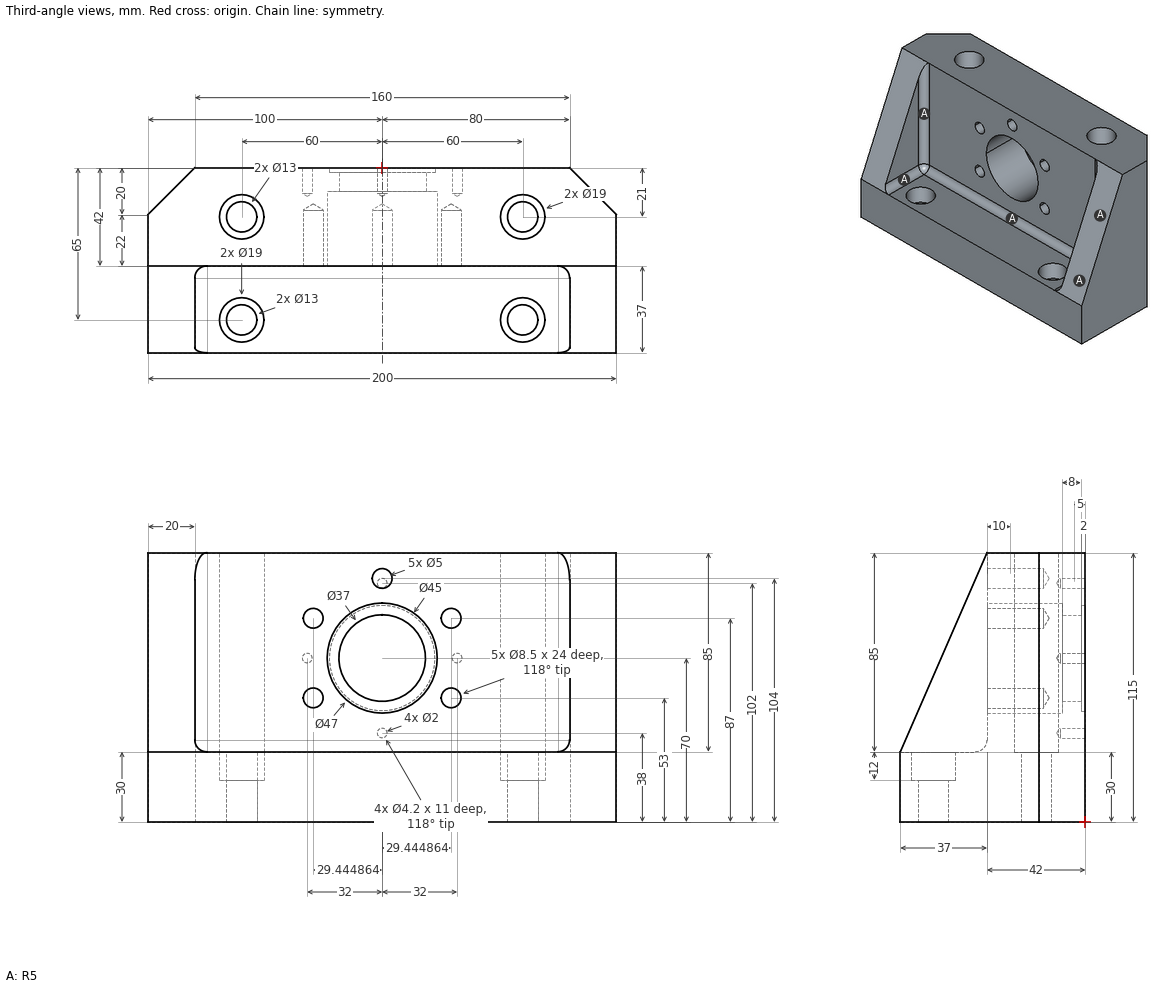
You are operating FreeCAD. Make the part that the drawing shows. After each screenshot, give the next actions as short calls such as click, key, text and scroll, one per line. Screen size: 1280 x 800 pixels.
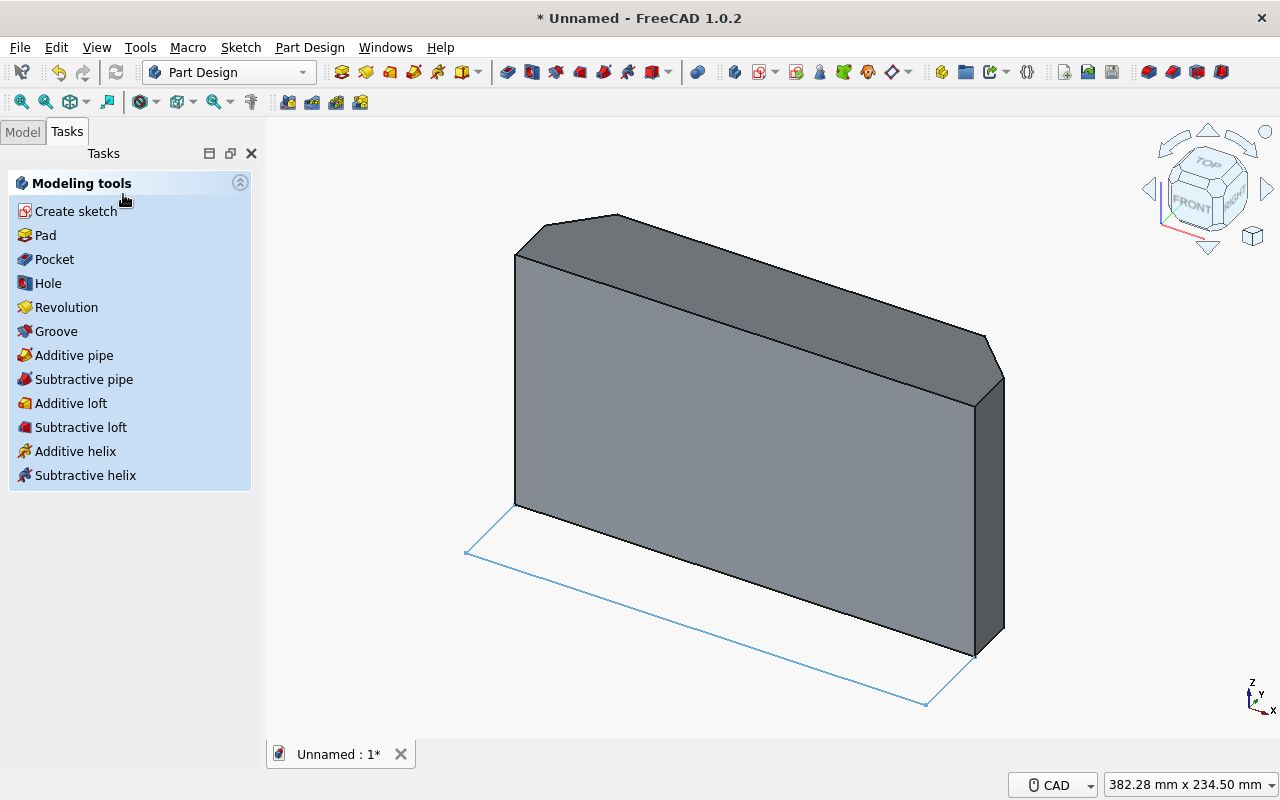
click(342, 72)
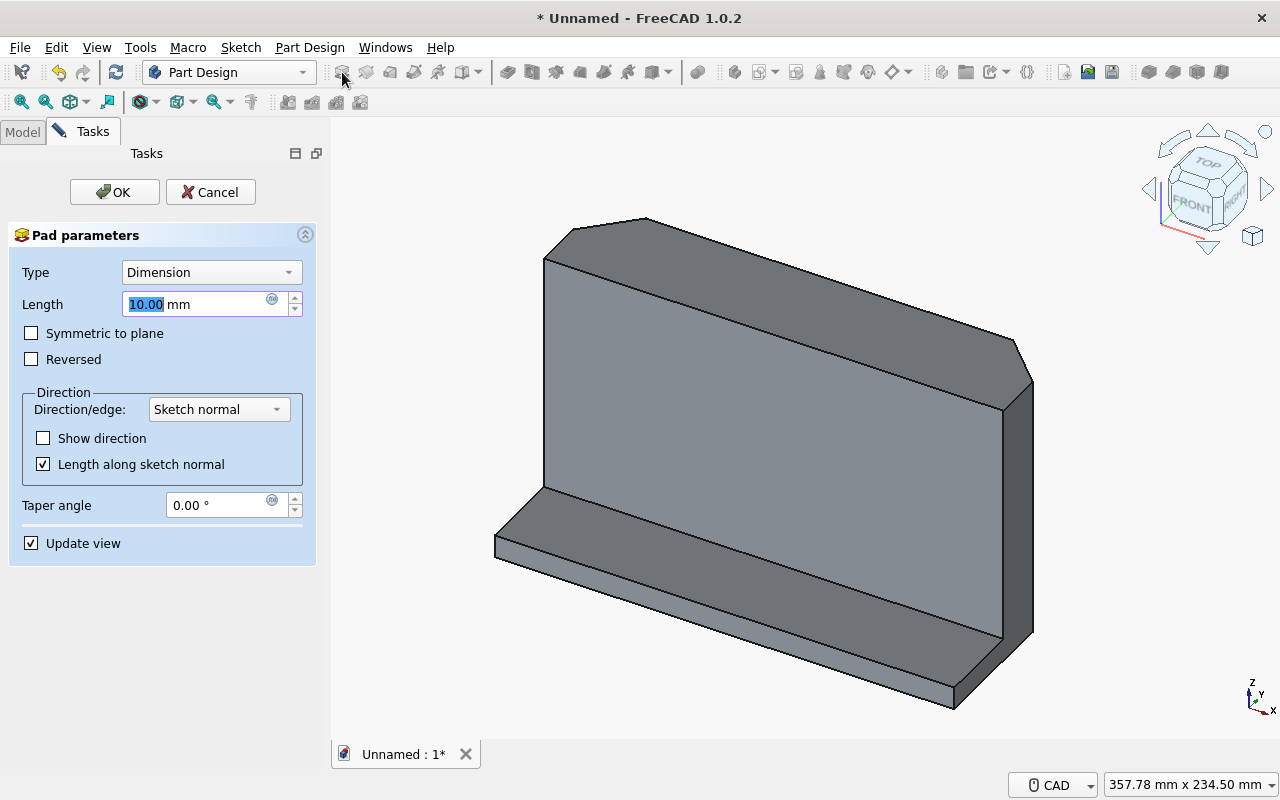
text(30)
key(Tab)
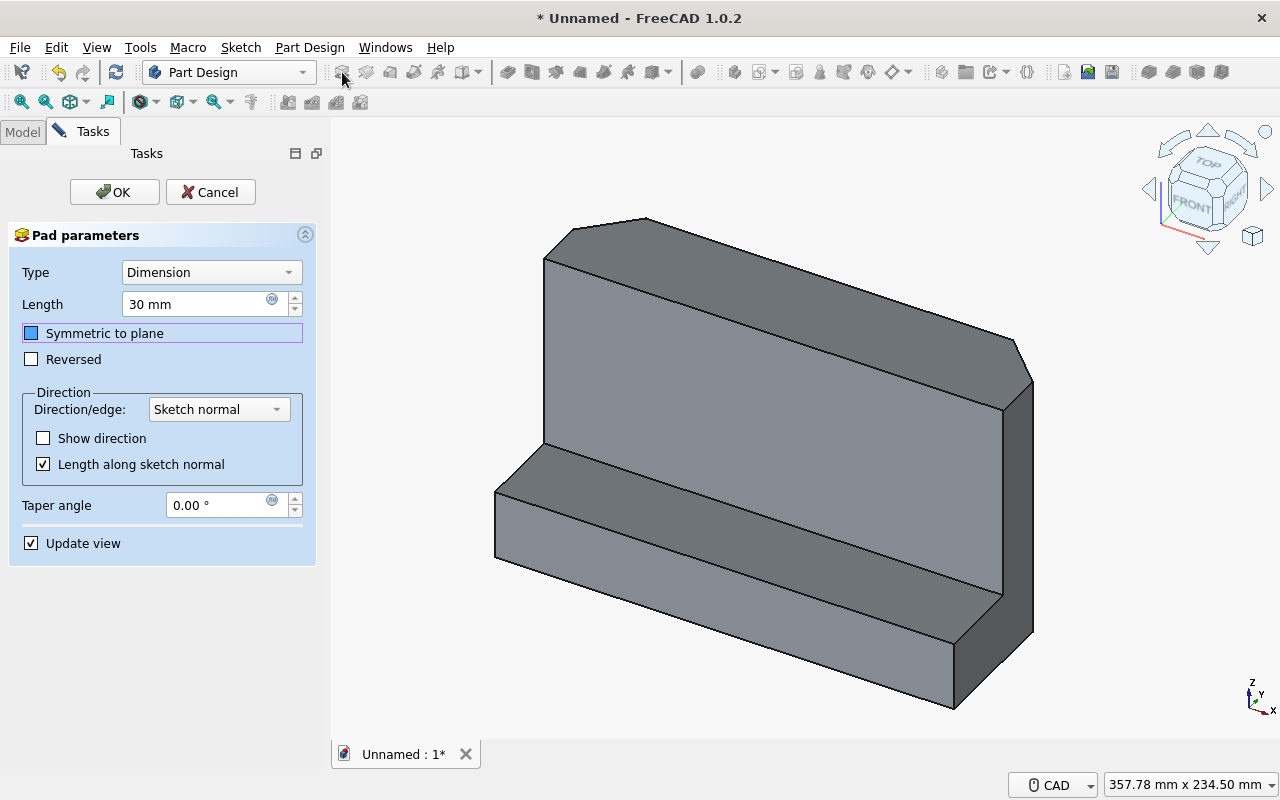
click(115, 192)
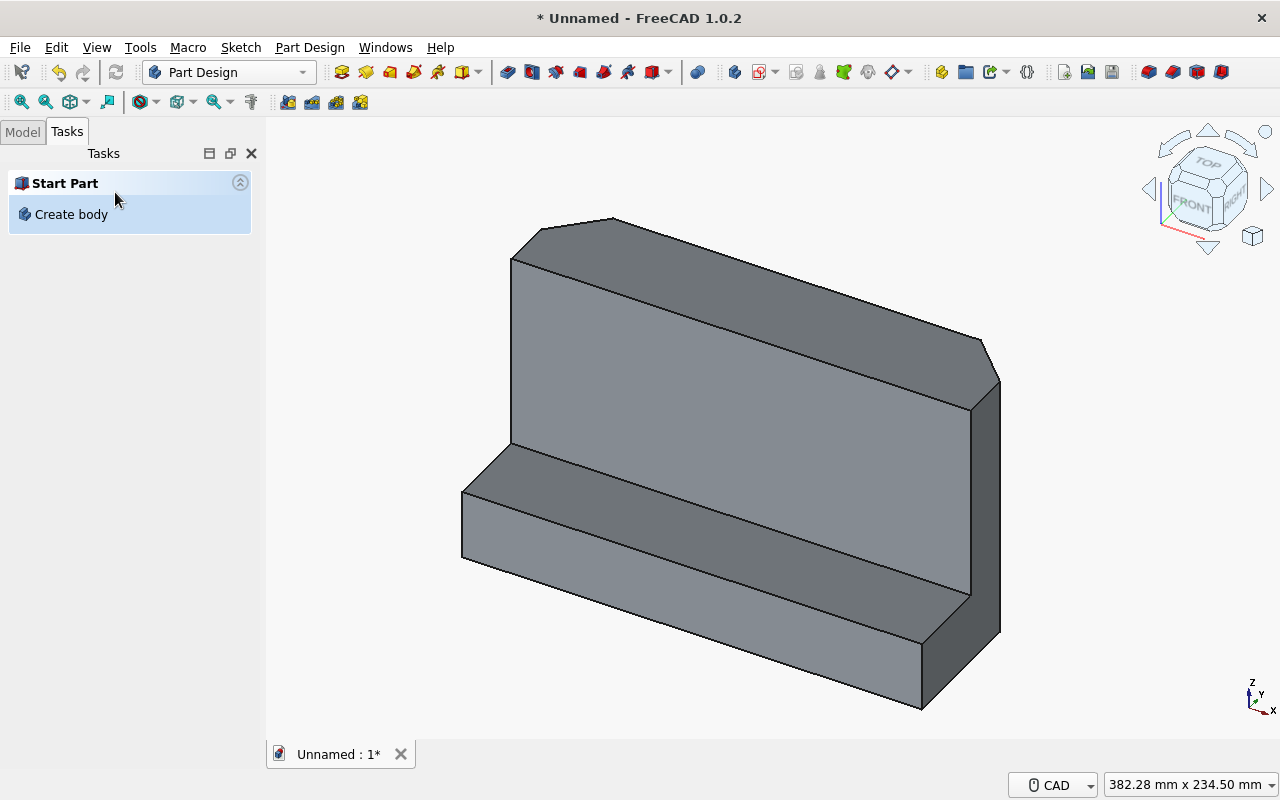
key(6)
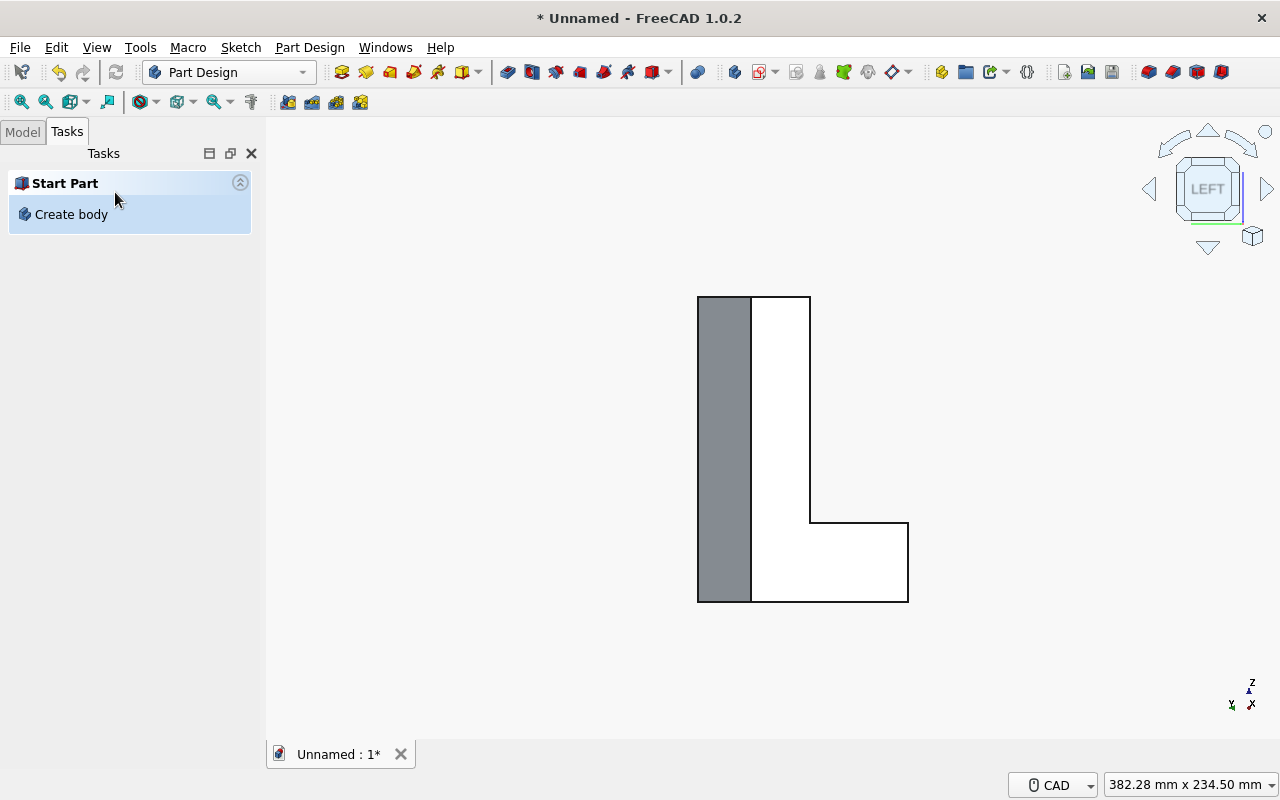
click(785, 536)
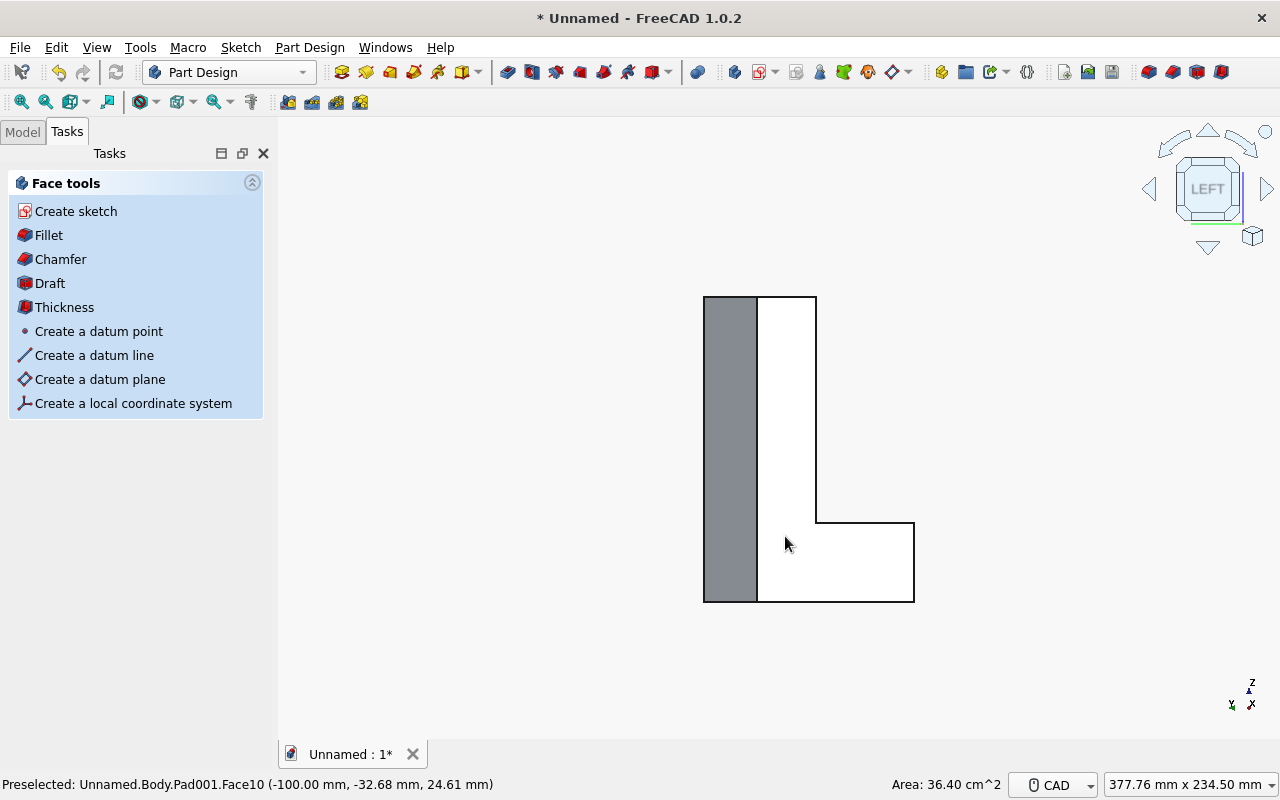
click(760, 72)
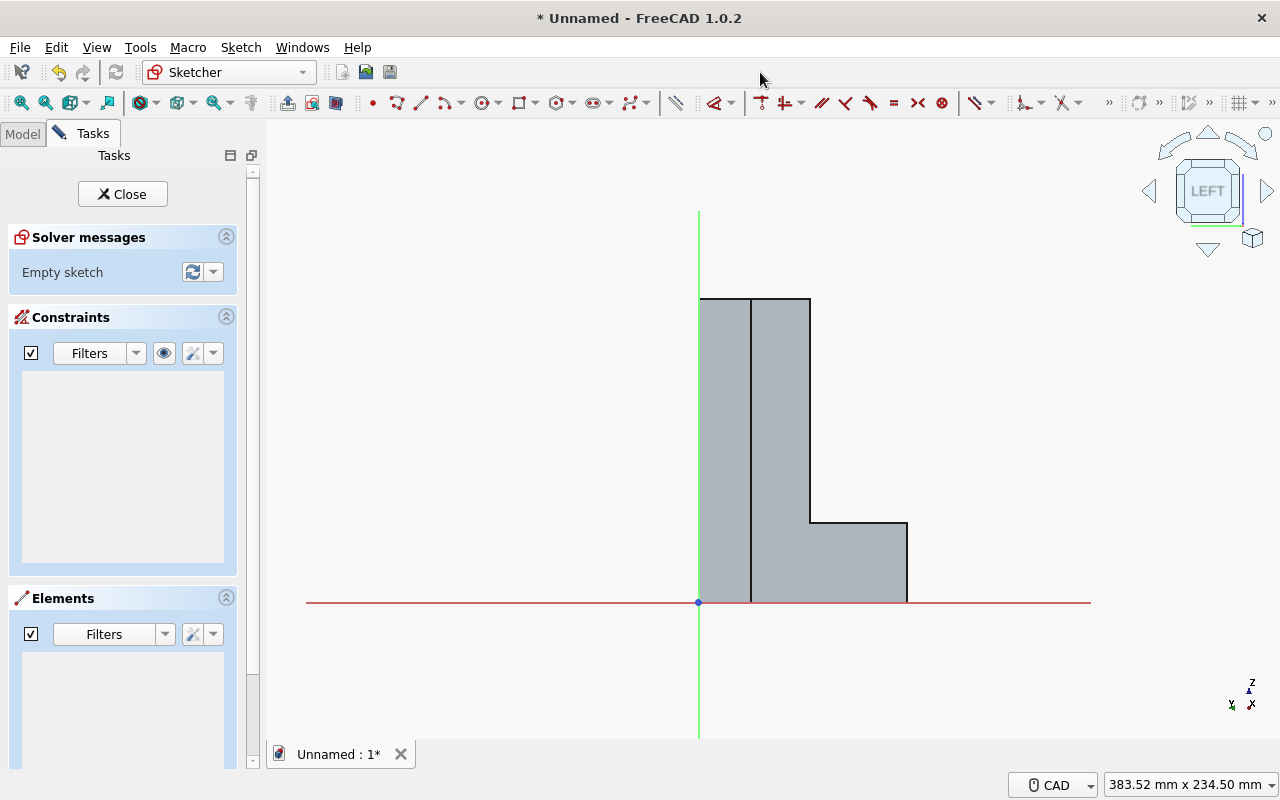
click(398, 104)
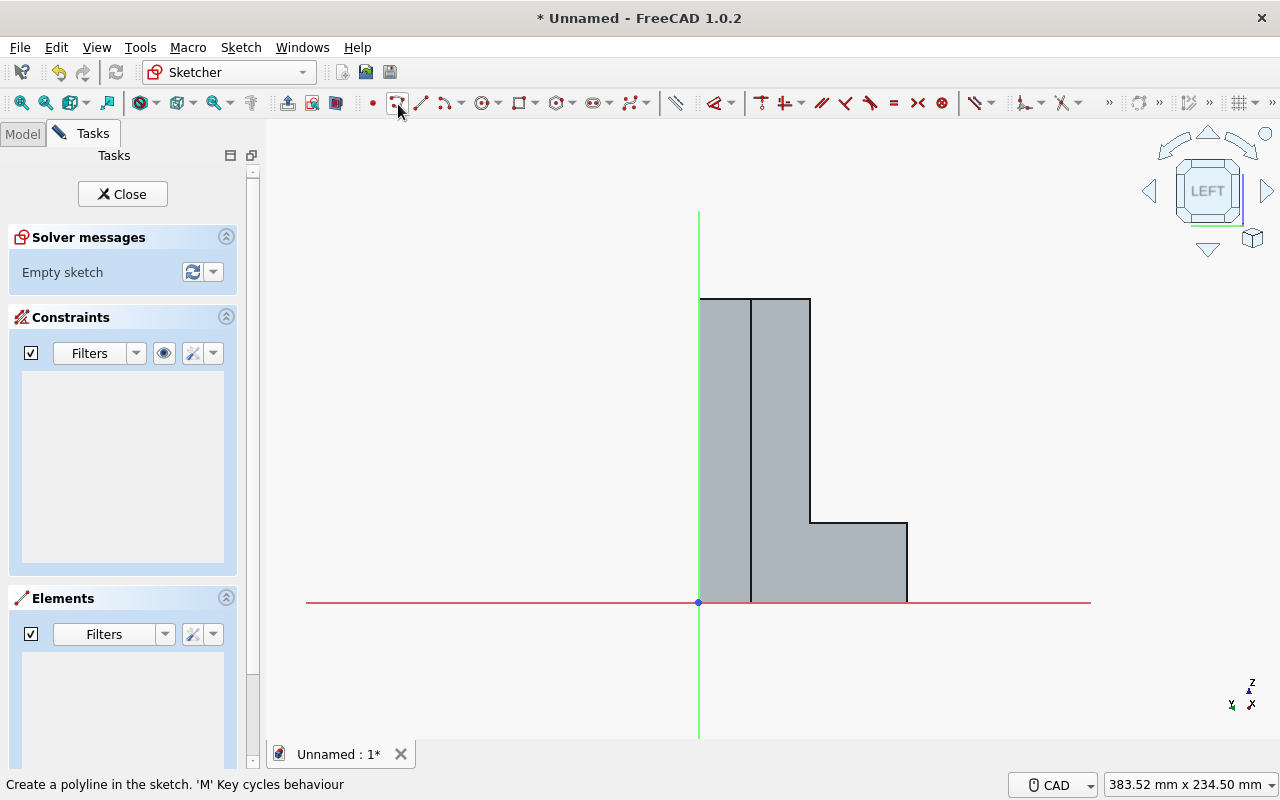
click(810, 523)
click(907, 523)
click(810, 299)
click(810, 524)
key(Escape)
key(Escape)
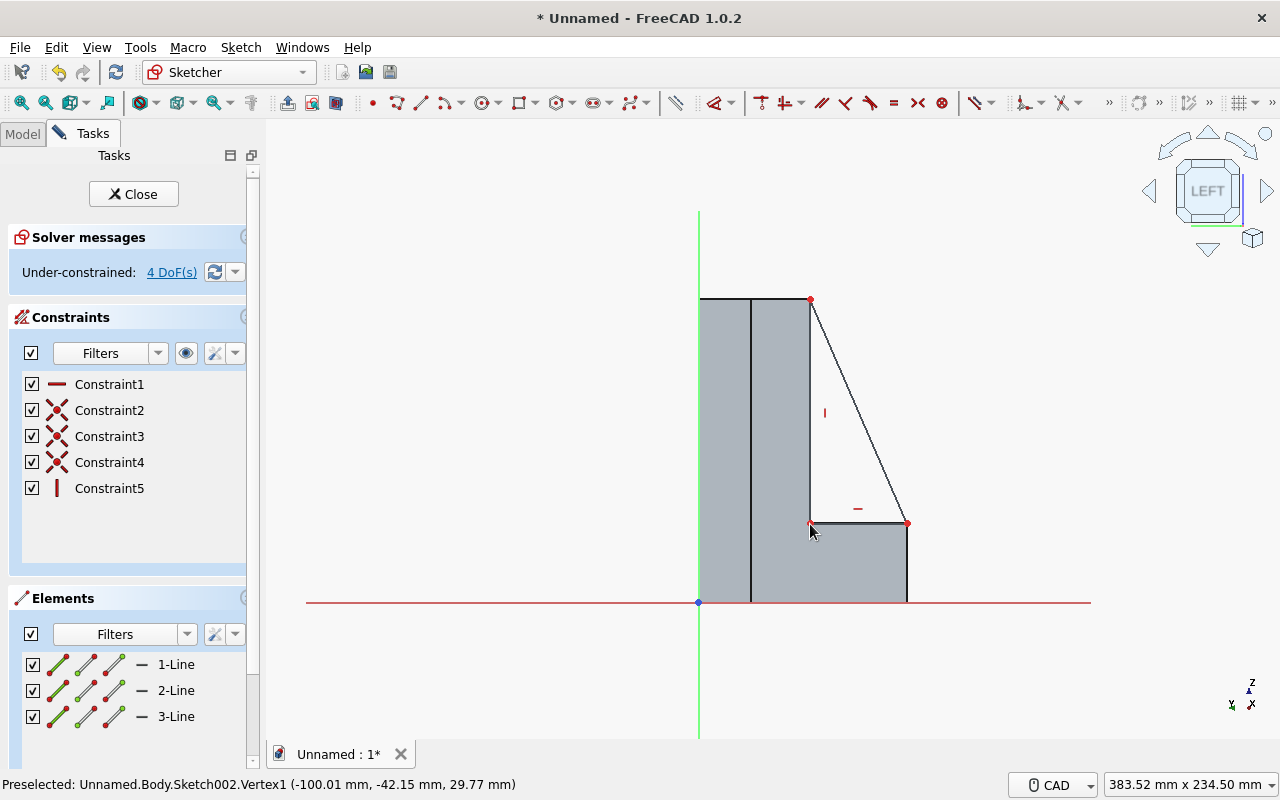
click(714, 104)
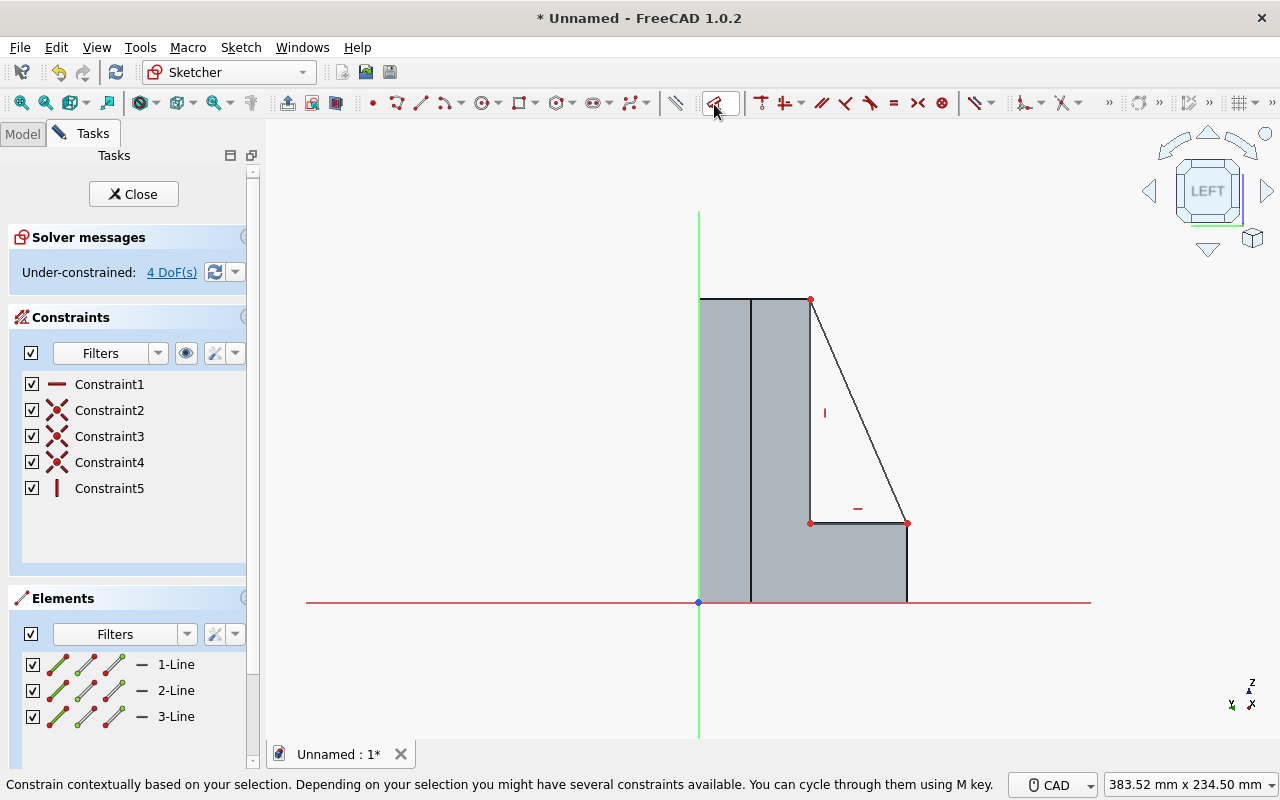
click(839, 524)
click(858, 558)